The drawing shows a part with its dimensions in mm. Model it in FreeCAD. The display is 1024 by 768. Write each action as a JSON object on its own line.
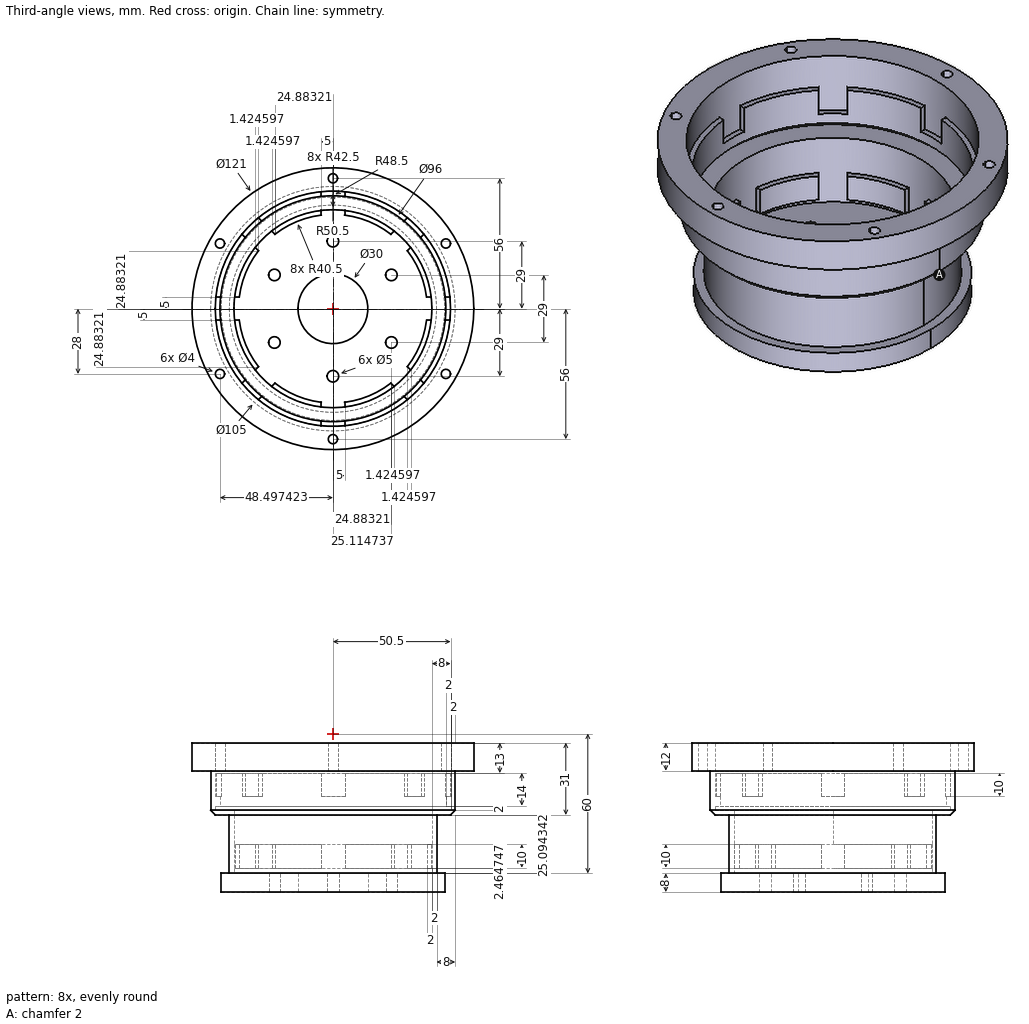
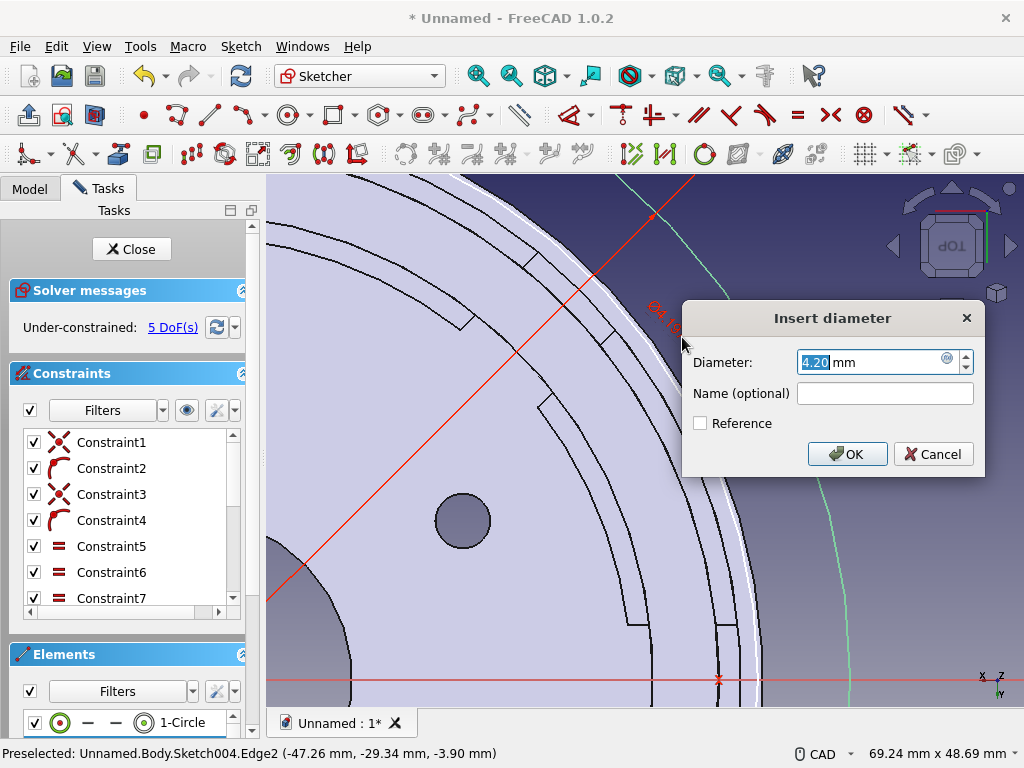
{"action": "type", "text": "4"}
{"action": "key", "text": "Return"}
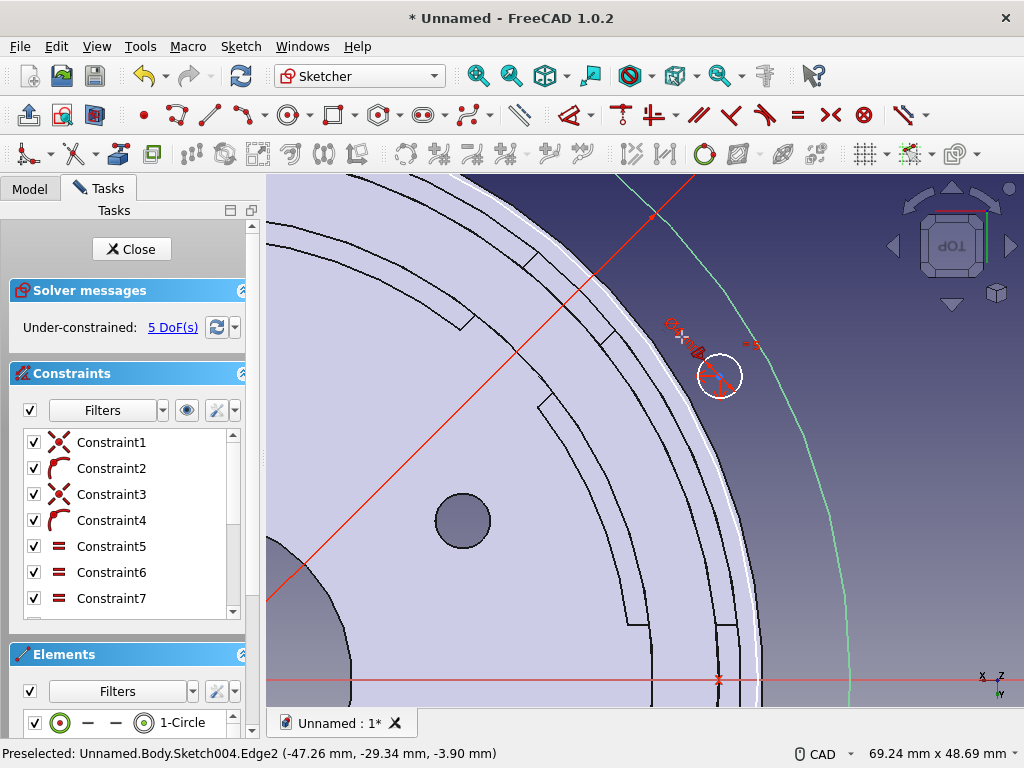
{"action": "scroll", "coordinate": [704, 362], "scroll_direction": "down", "scroll_amount": 7}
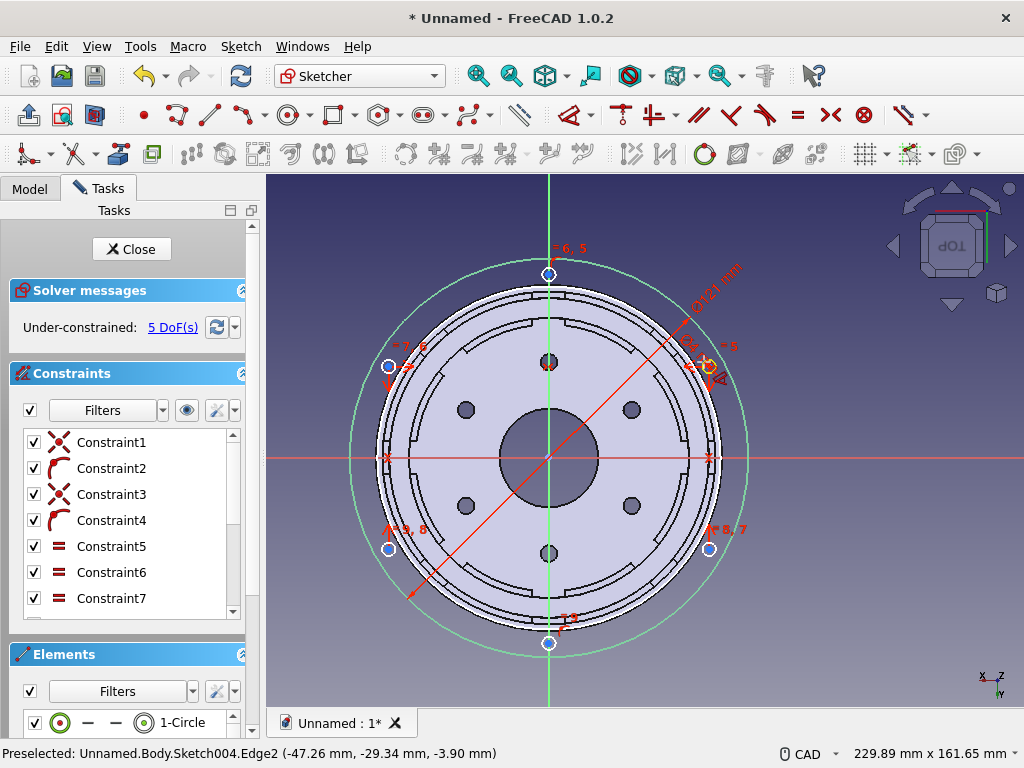
{"action": "left_click", "coordinate": [676, 341]}
{"action": "left_click", "coordinate": [764, 385]}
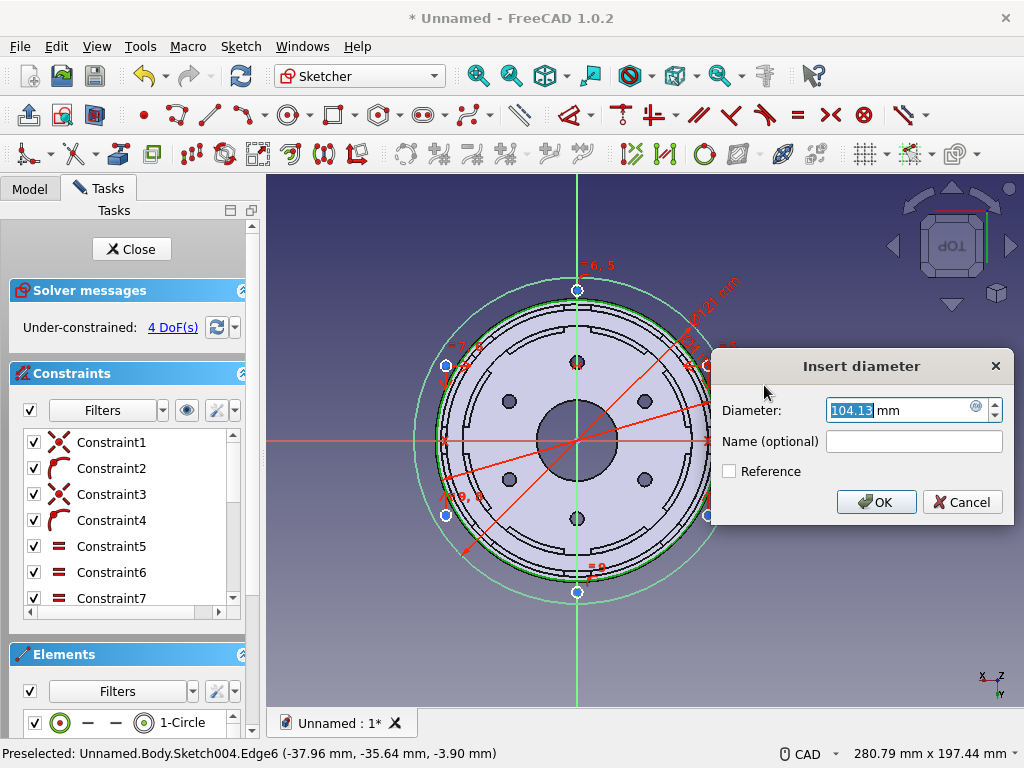
{"action": "type", "text": "105"}
{"action": "key", "text": "Return"}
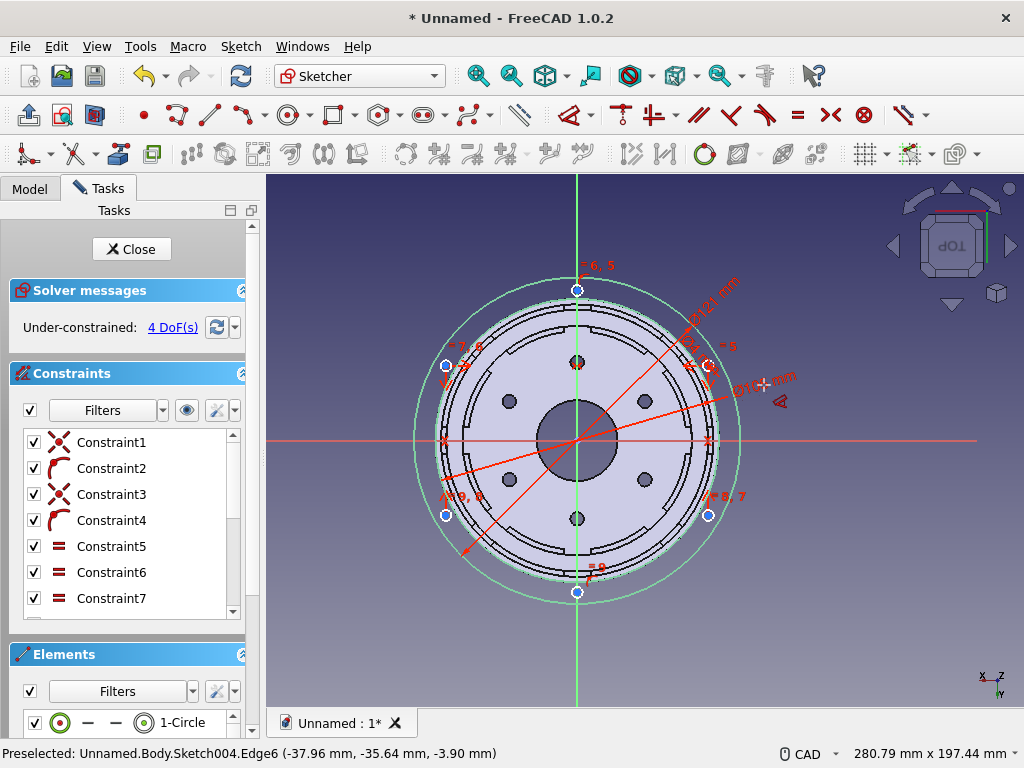
{"action": "left_click", "coordinate": [708, 366]}
{"action": "left_click", "coordinate": [543, 403]}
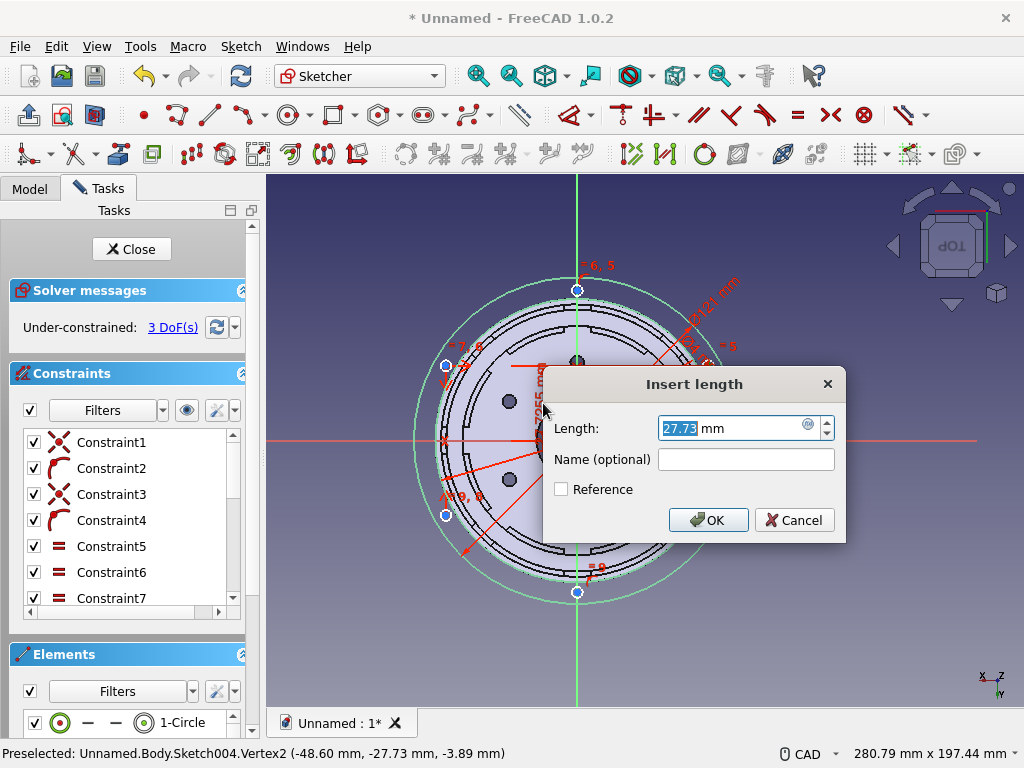
{"action": "type", "text": "28"}
{"action": "key", "text": "Return"}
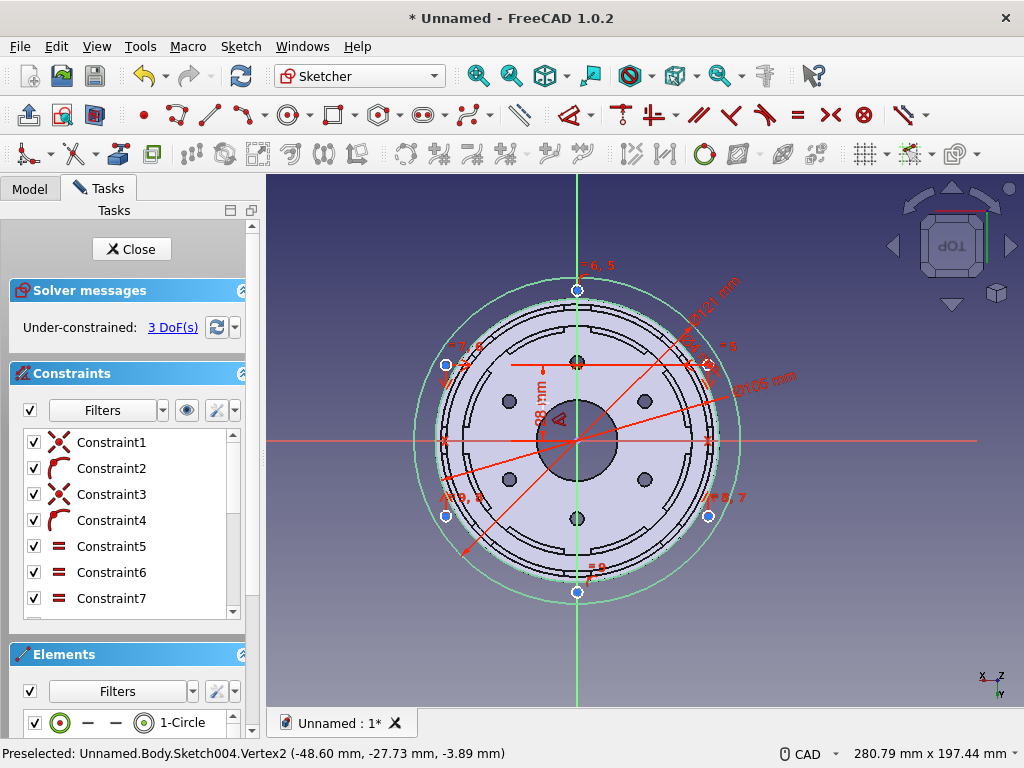
{"action": "left_click", "coordinate": [577, 290]}
{"action": "left_click", "coordinate": [611, 366]}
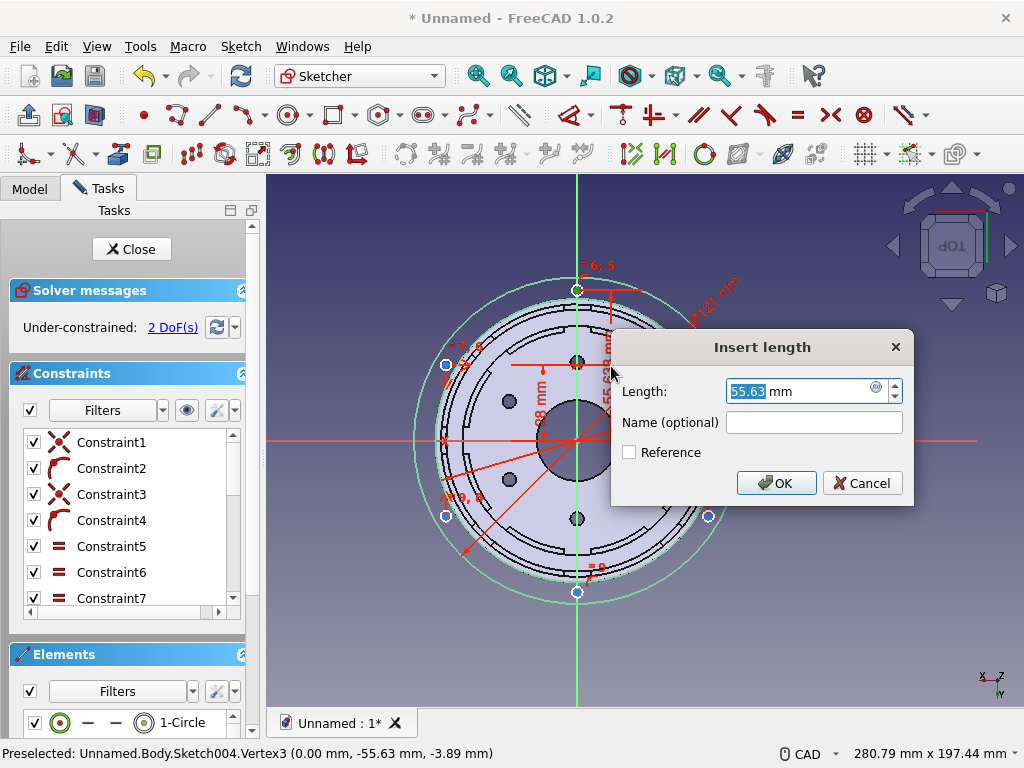
{"action": "type", "text": "56"}
{"action": "key", "text": "Return"}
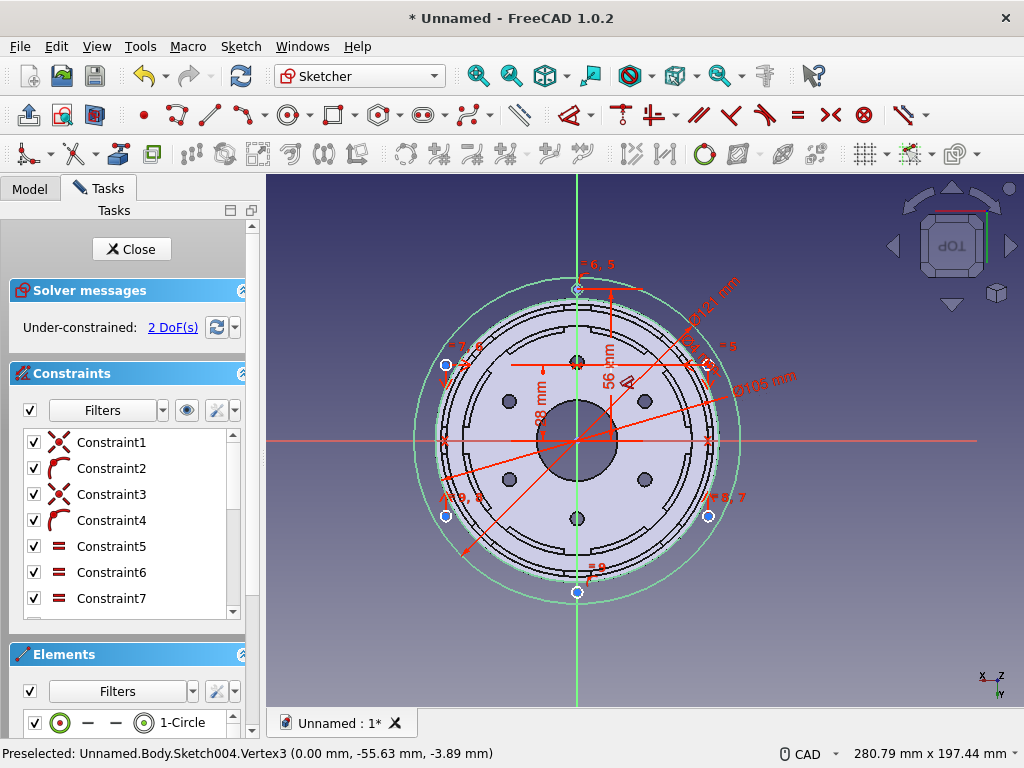
{"action": "left_click", "coordinate": [577, 592]}
{"action": "left_click", "coordinate": [611, 516]}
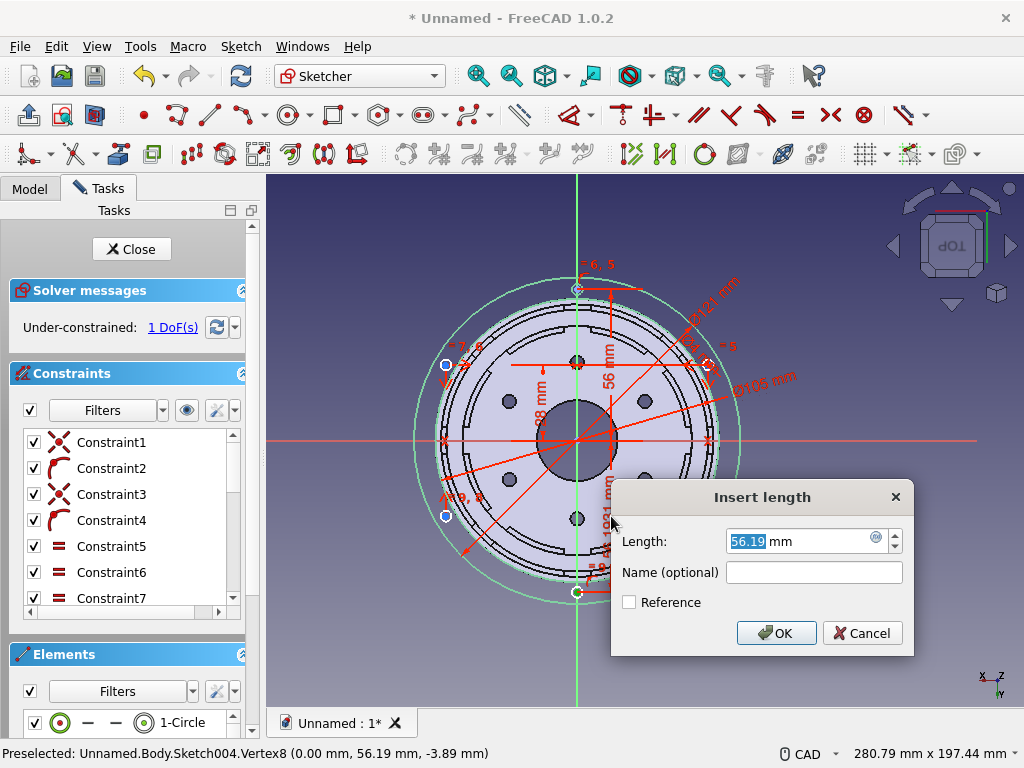
{"action": "type", "text": "56"}
{"action": "key", "text": "Return"}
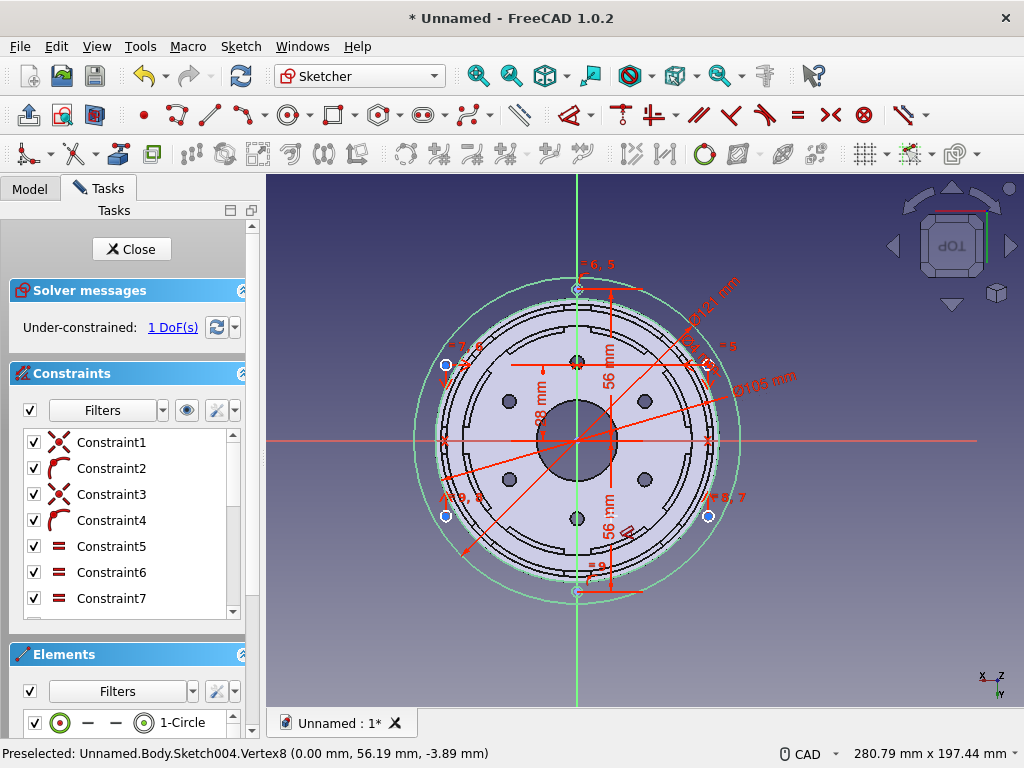
{"action": "left_click", "coordinate": [708, 365]}
{"action": "left_click", "coordinate": [643, 331]}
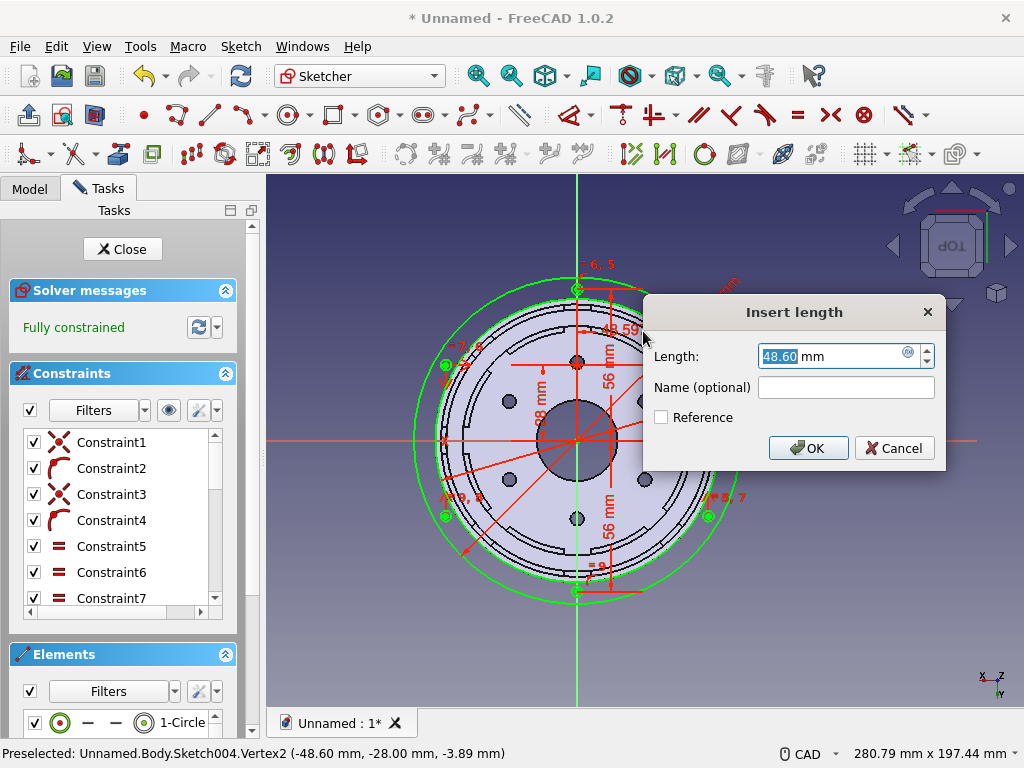
{"action": "type", "text": "48.497423"}
{"action": "key", "text": "Return"}
{"action": "key", "text": "Escape"}